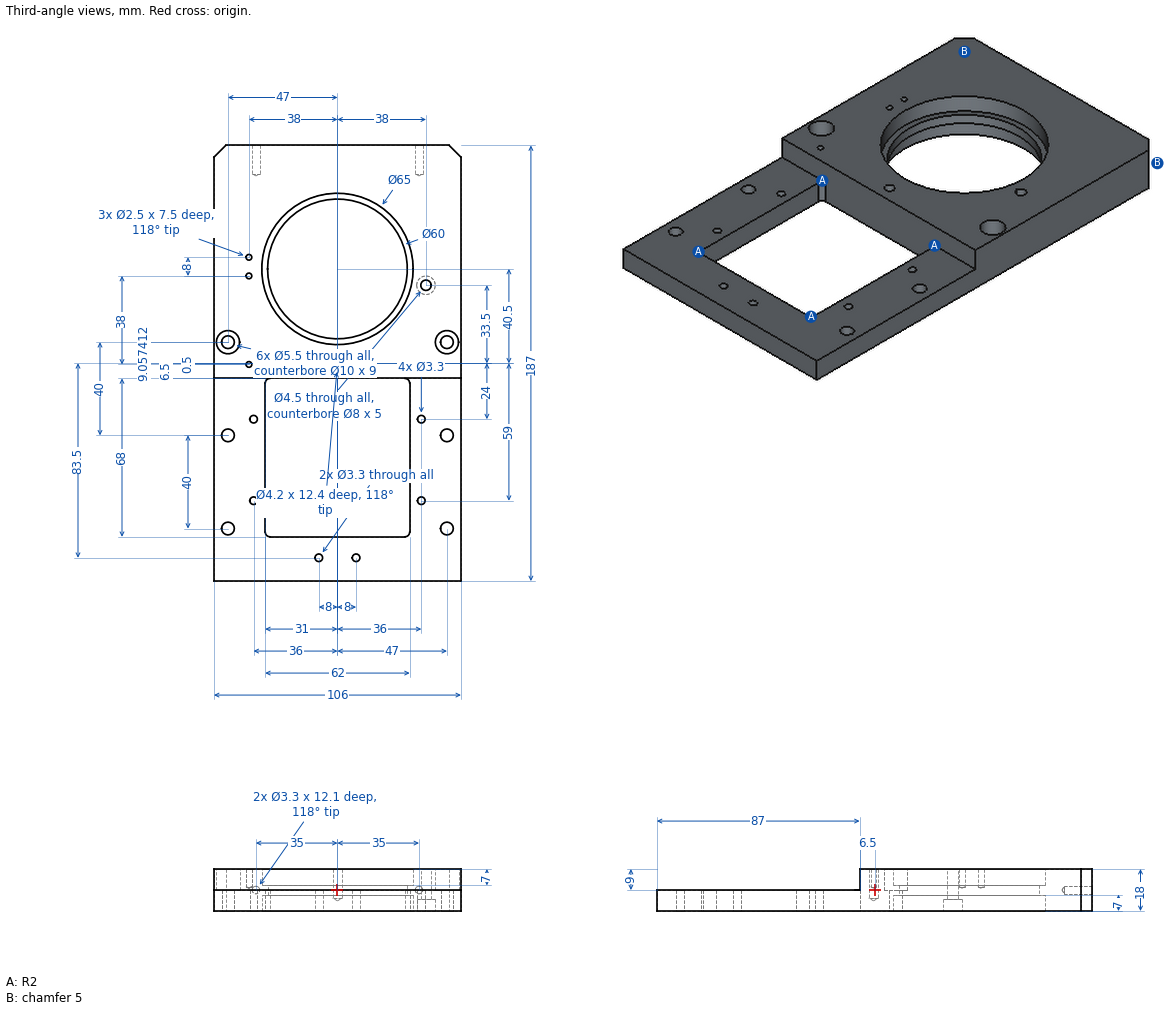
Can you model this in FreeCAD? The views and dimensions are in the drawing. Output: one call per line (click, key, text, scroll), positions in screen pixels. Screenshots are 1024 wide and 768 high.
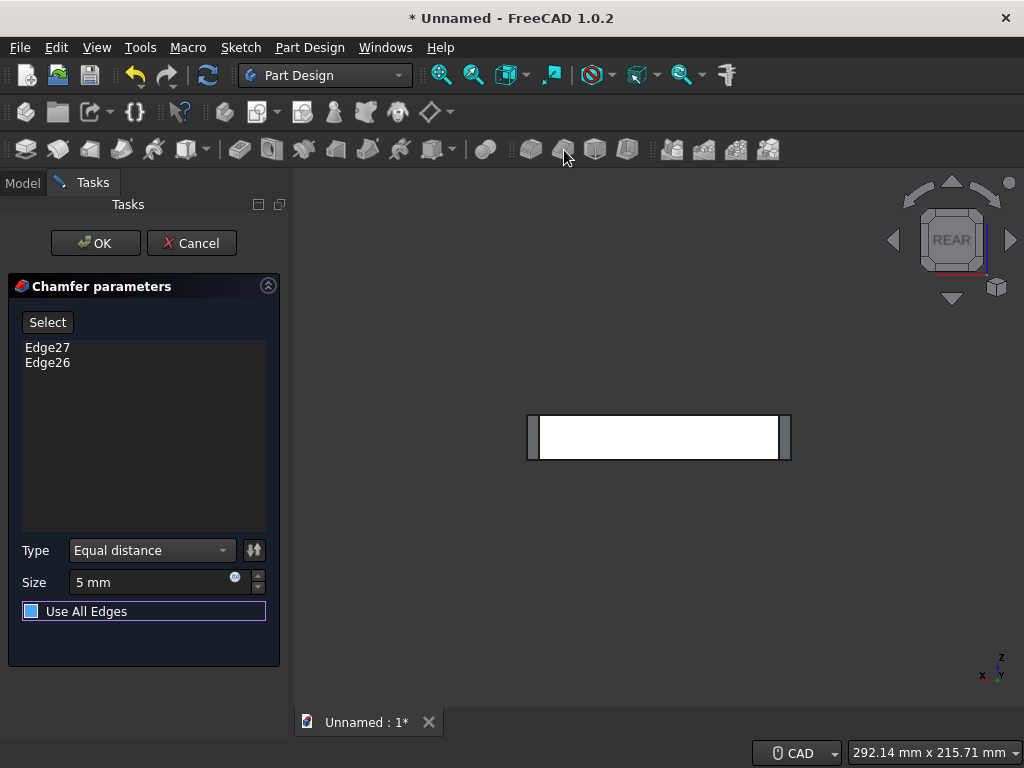
click(96, 243)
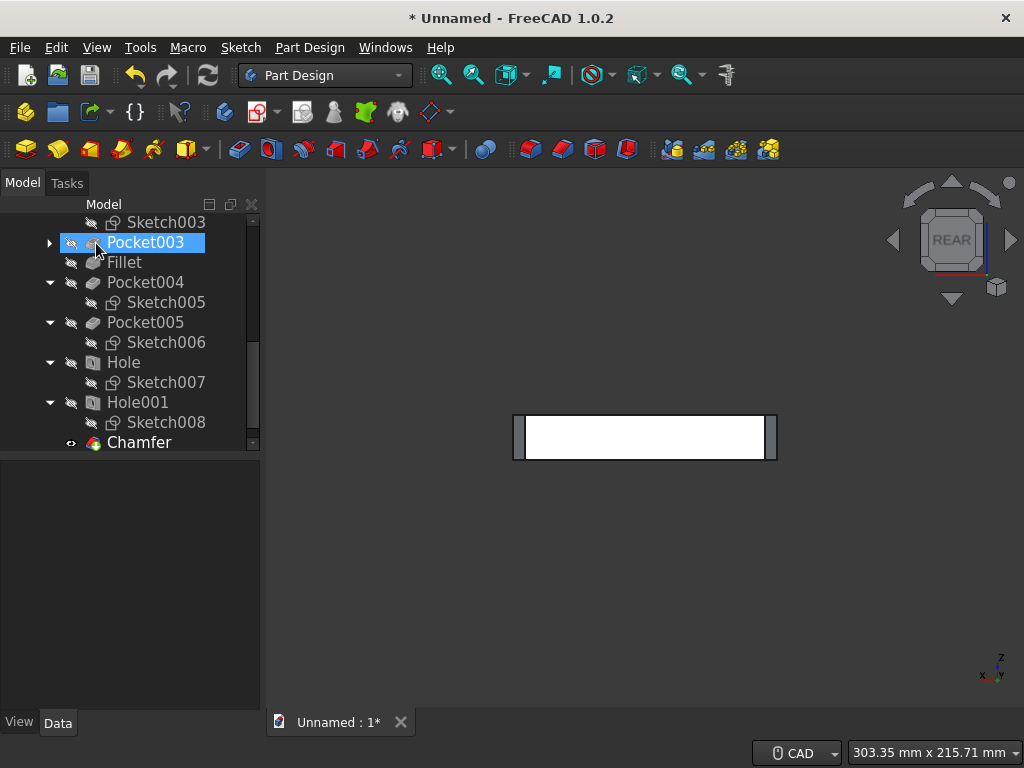
click(442, 76)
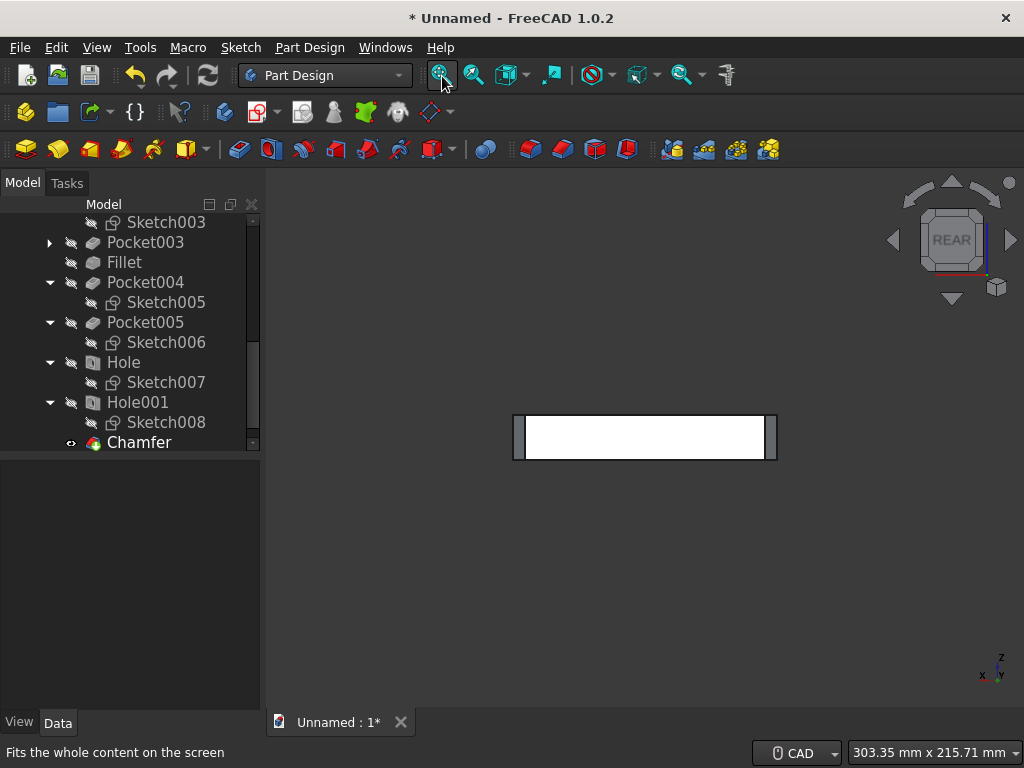
key(5)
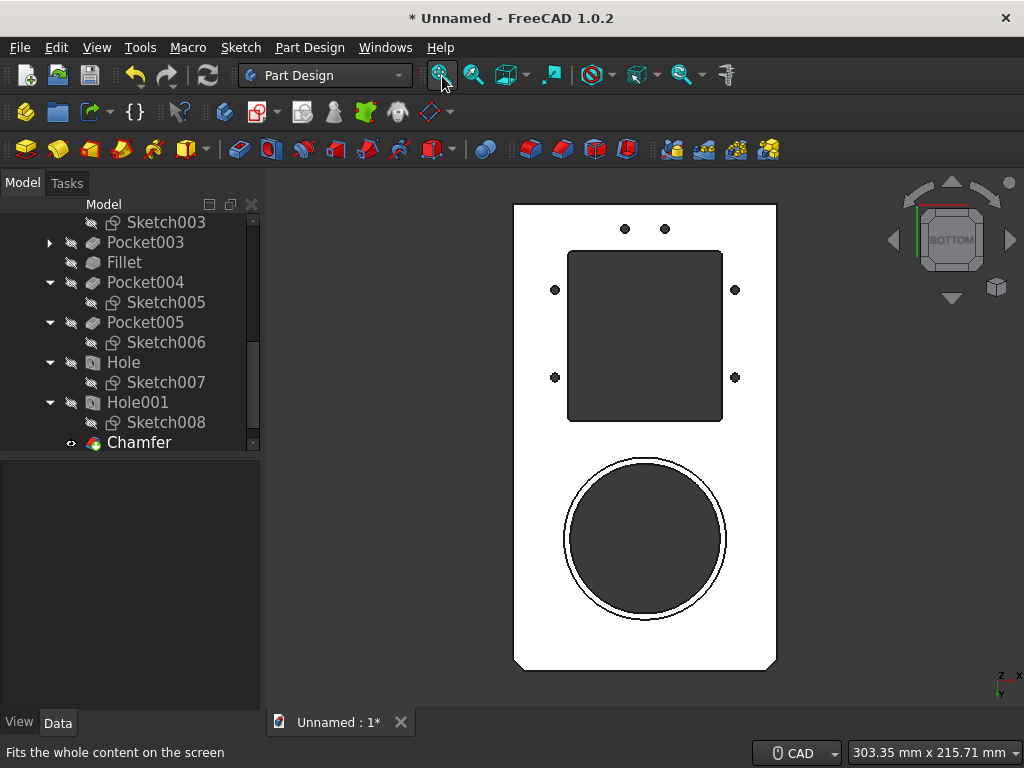
click(721, 637)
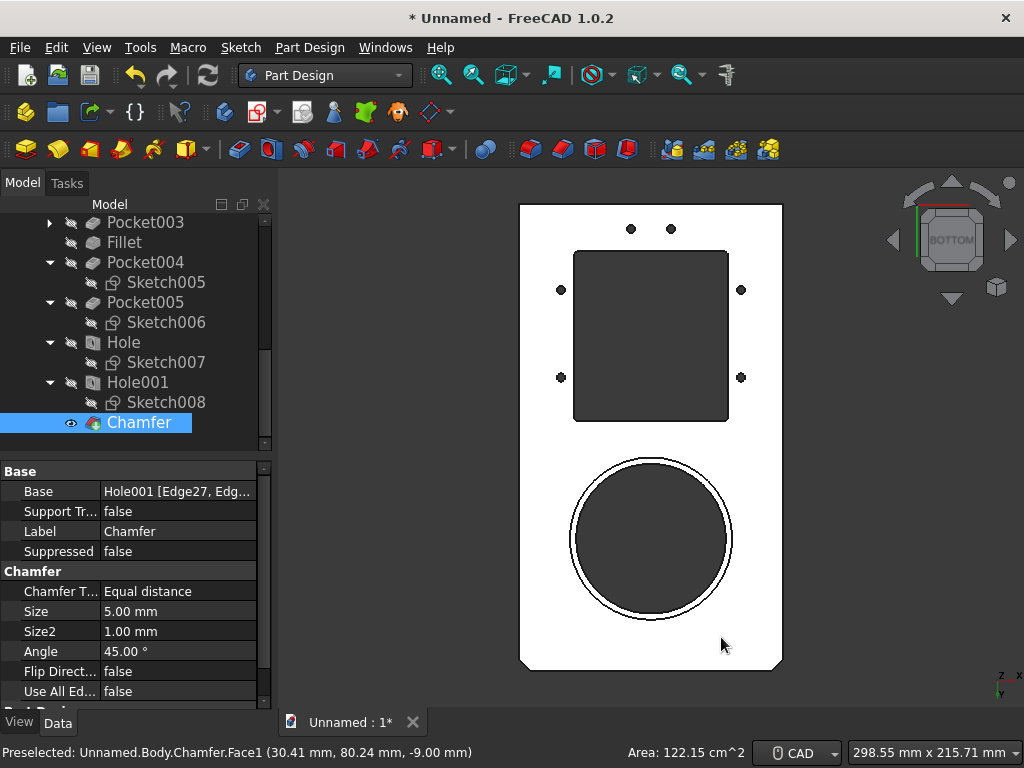
click(258, 112)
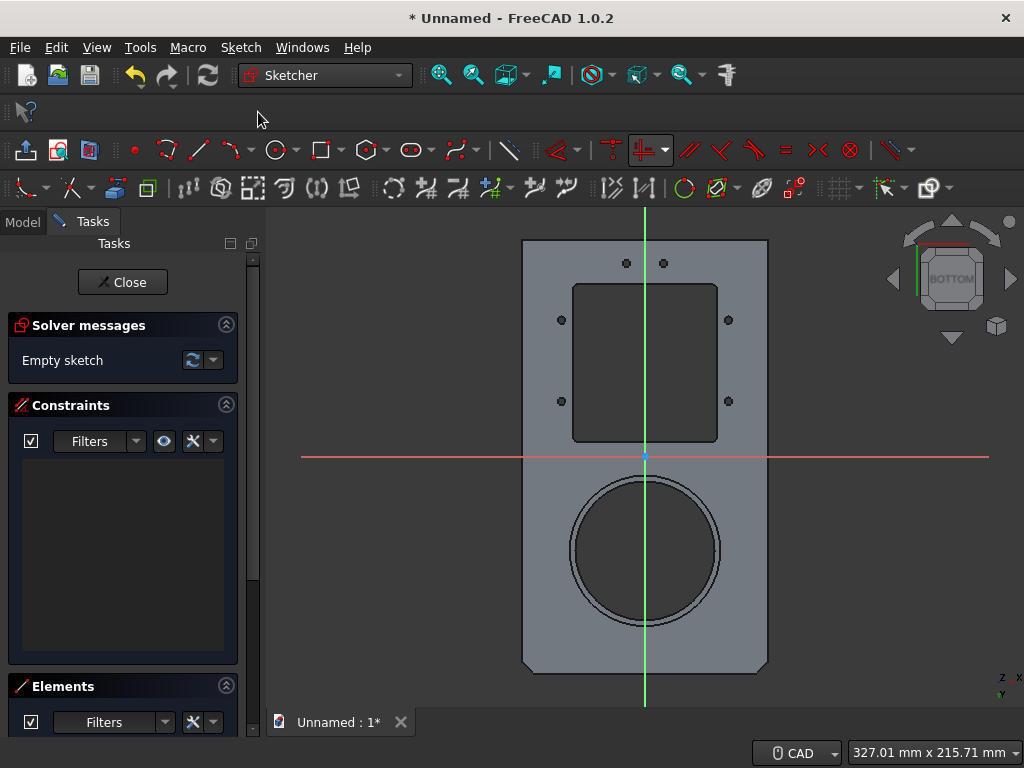
scroll(741, 539, up, 15)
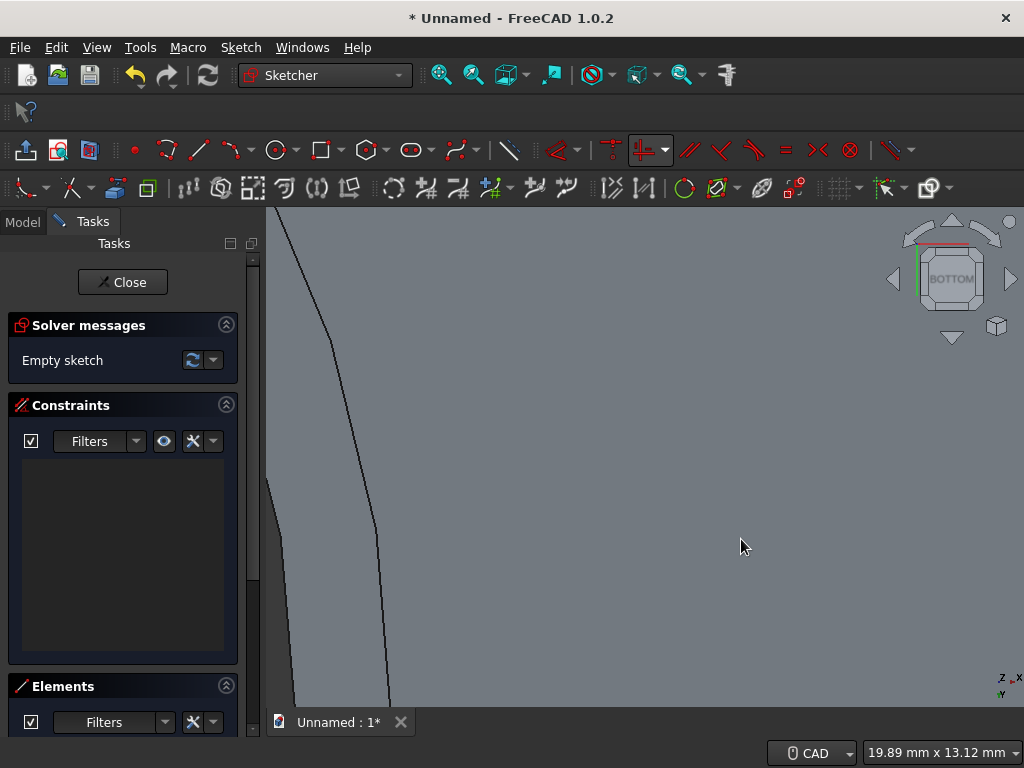
scroll(557, 402, up, 2)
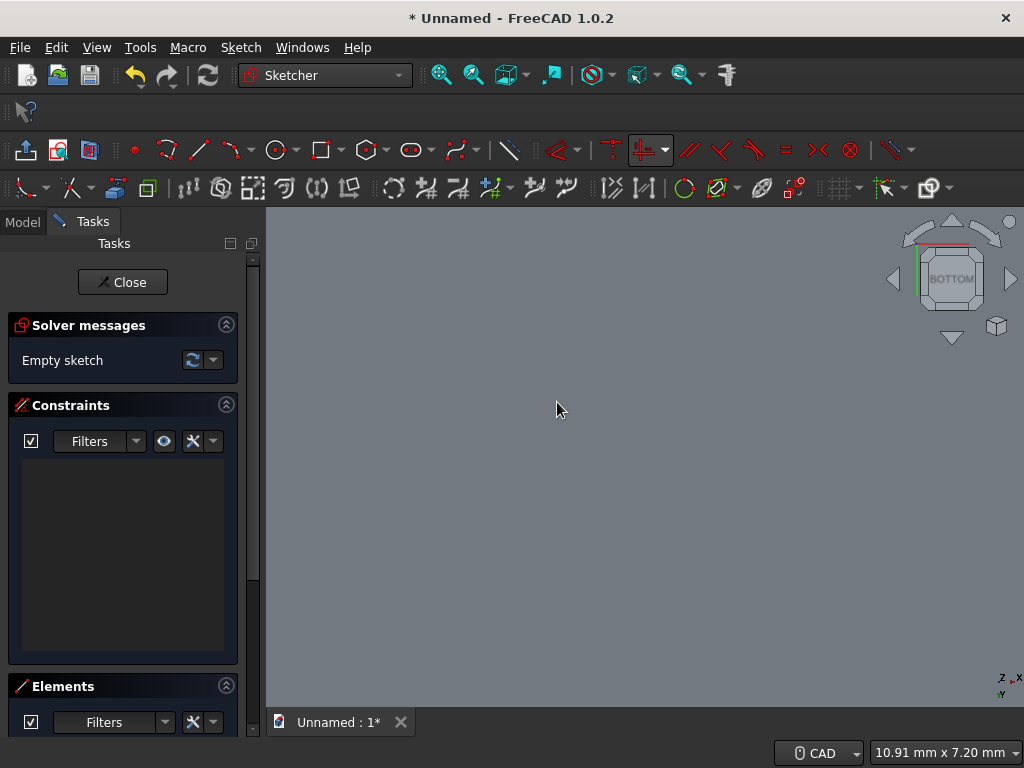
click(276, 150)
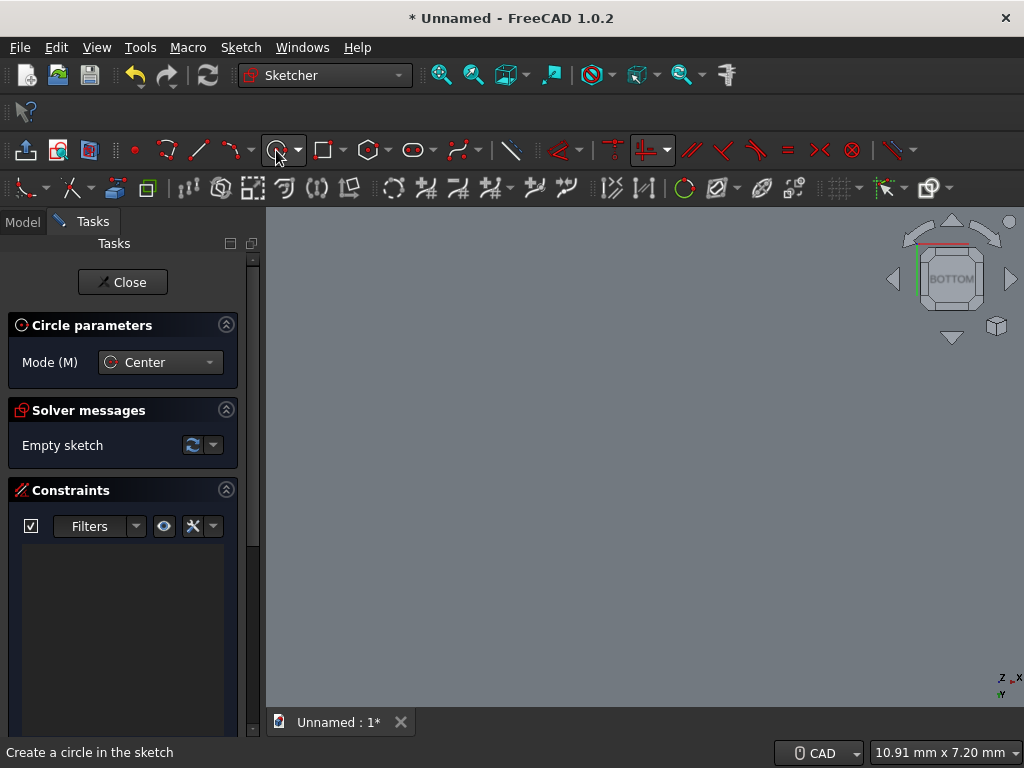
click(576, 457)
click(687, 346)
key(Escape)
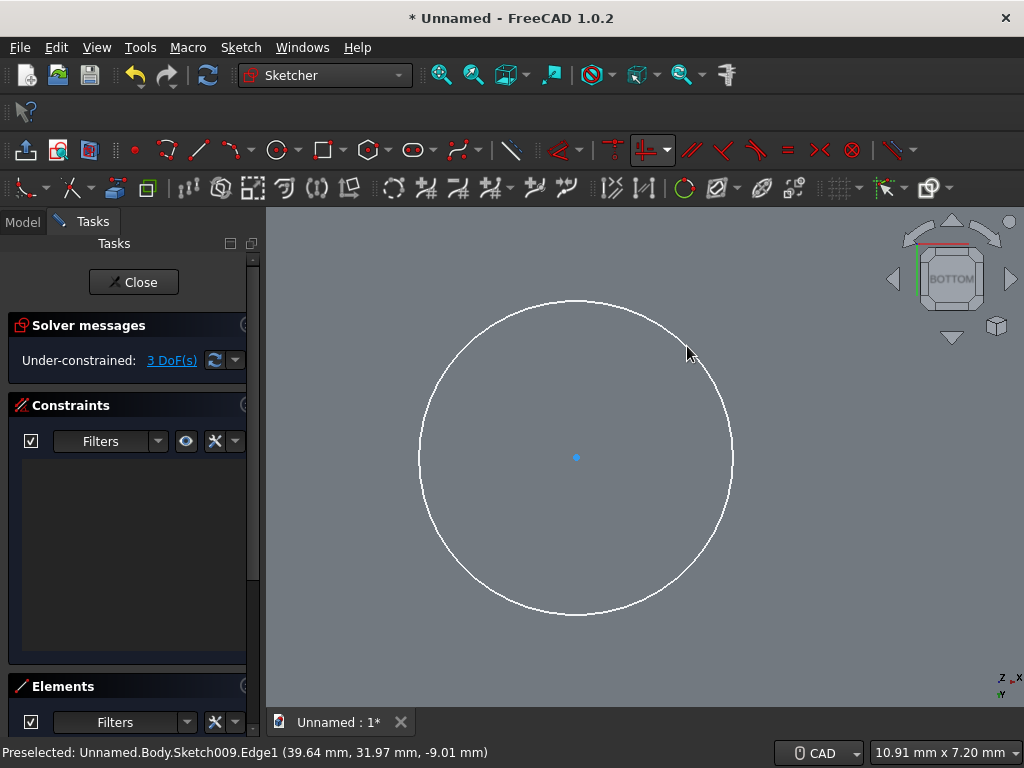
click(558, 150)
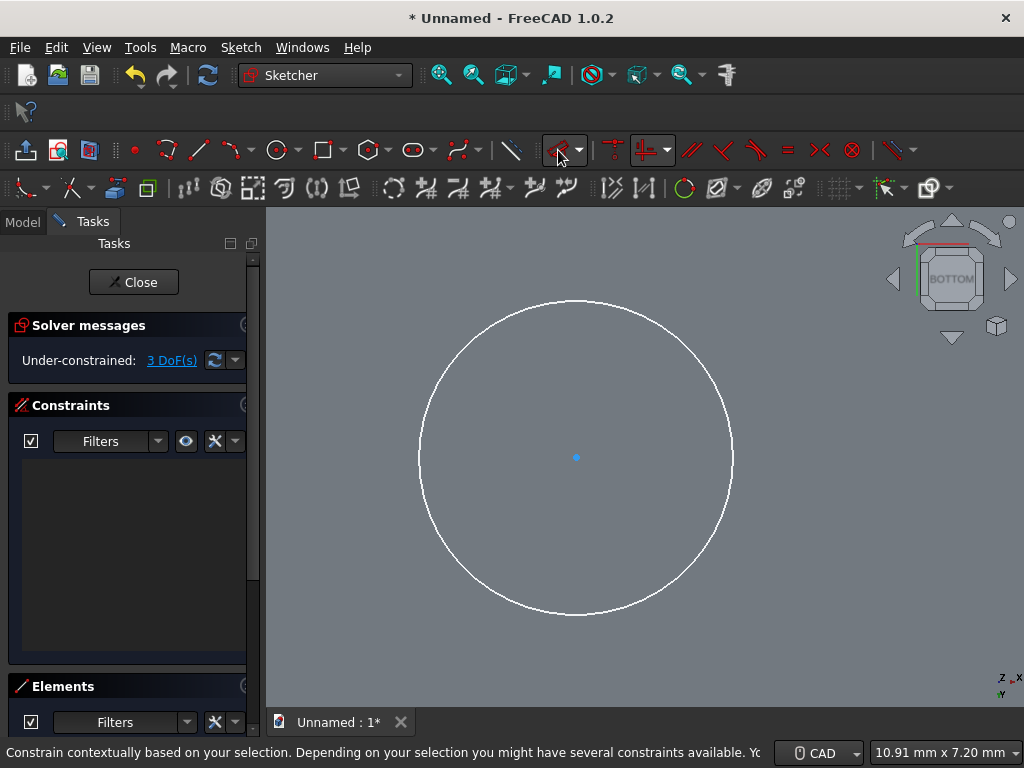
click(687, 347)
click(710, 324)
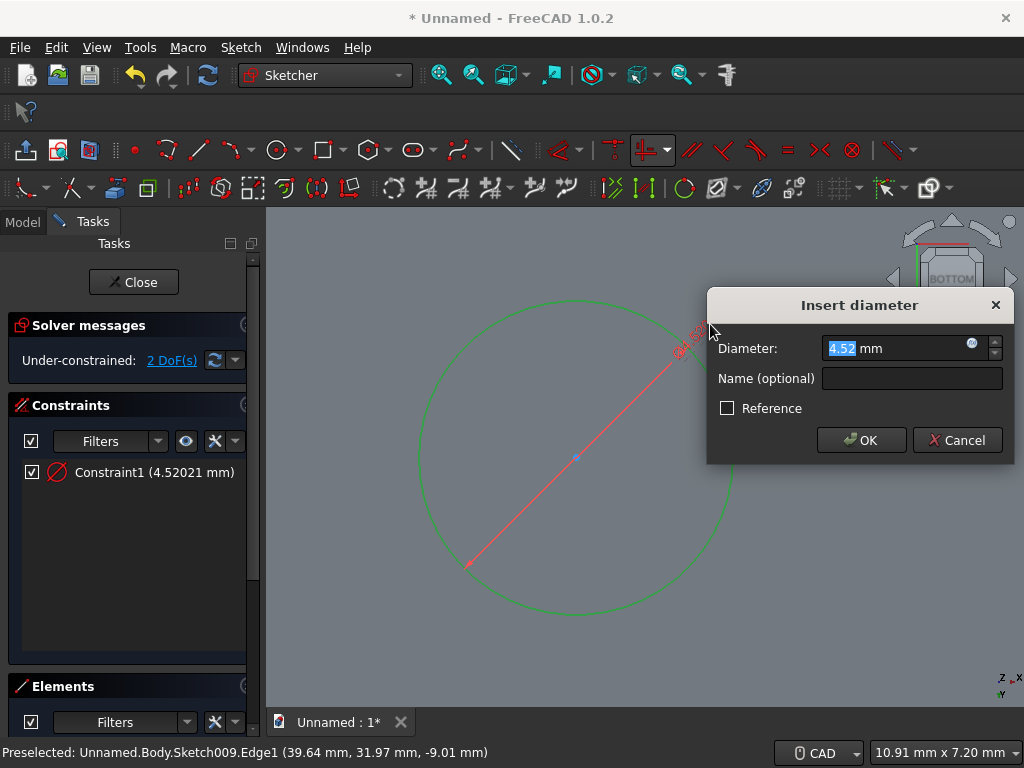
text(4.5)
key(Return)